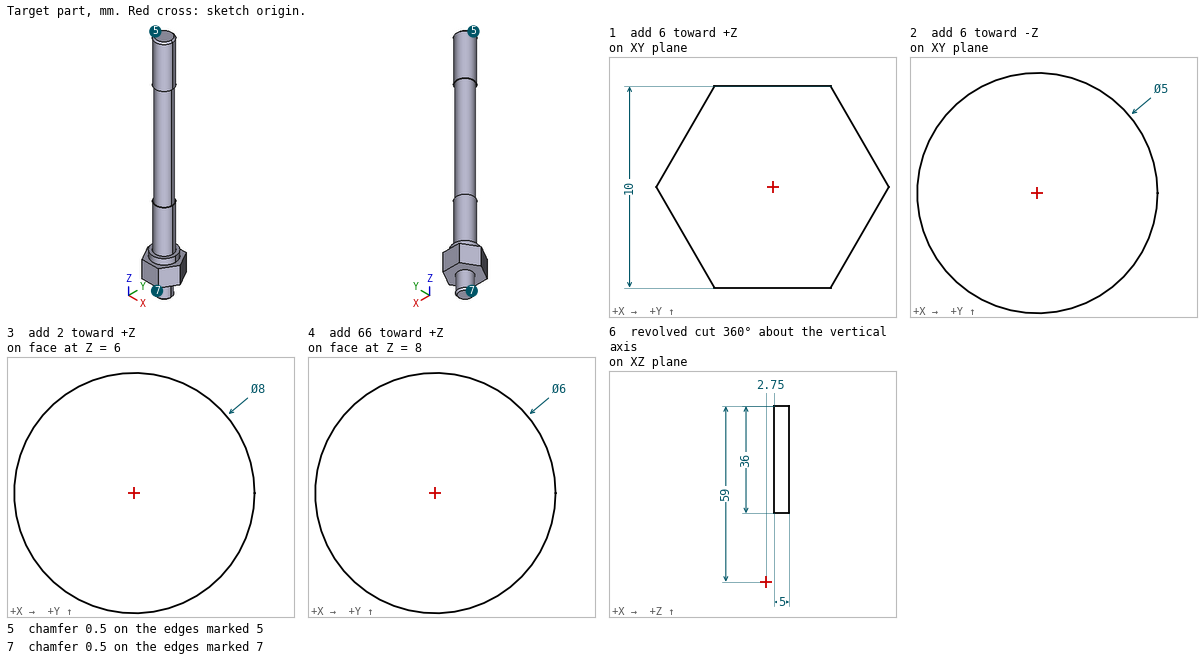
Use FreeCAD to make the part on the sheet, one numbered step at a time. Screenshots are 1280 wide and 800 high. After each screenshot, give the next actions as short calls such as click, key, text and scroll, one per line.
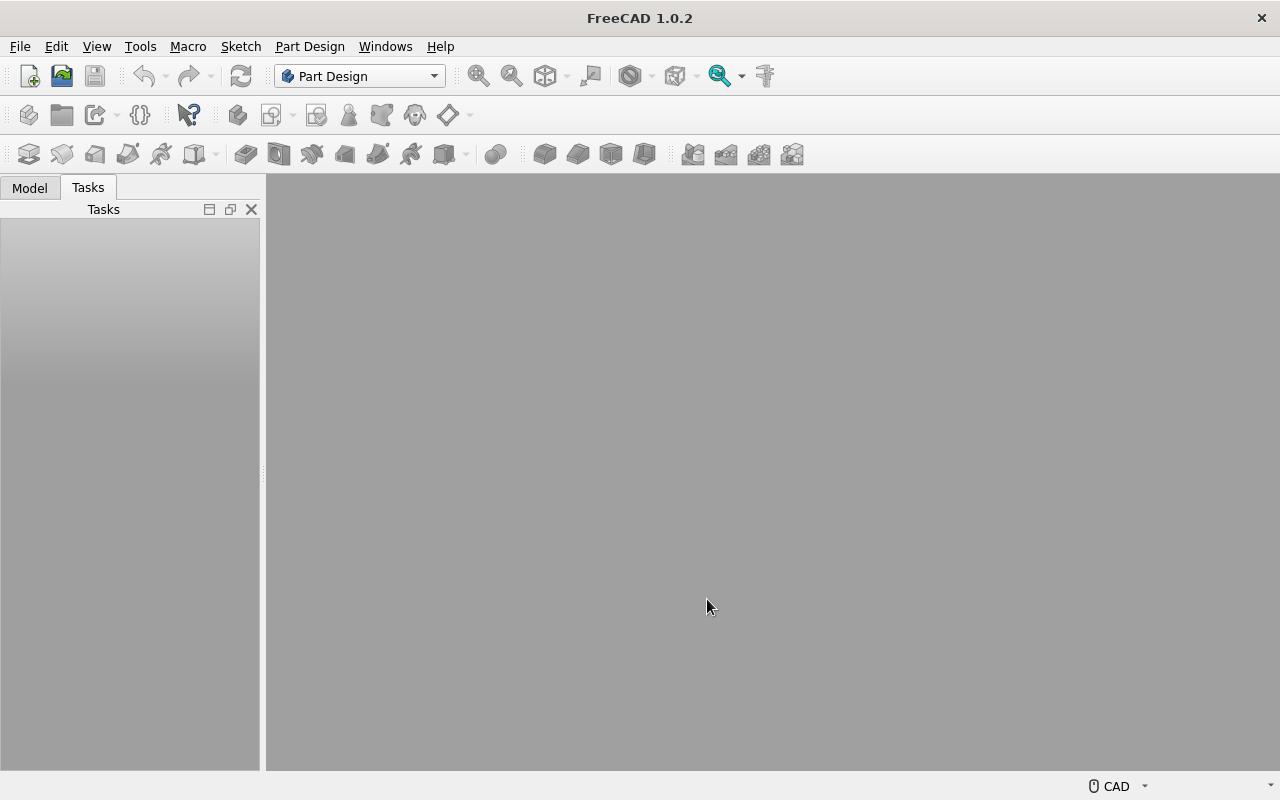
click(29, 76)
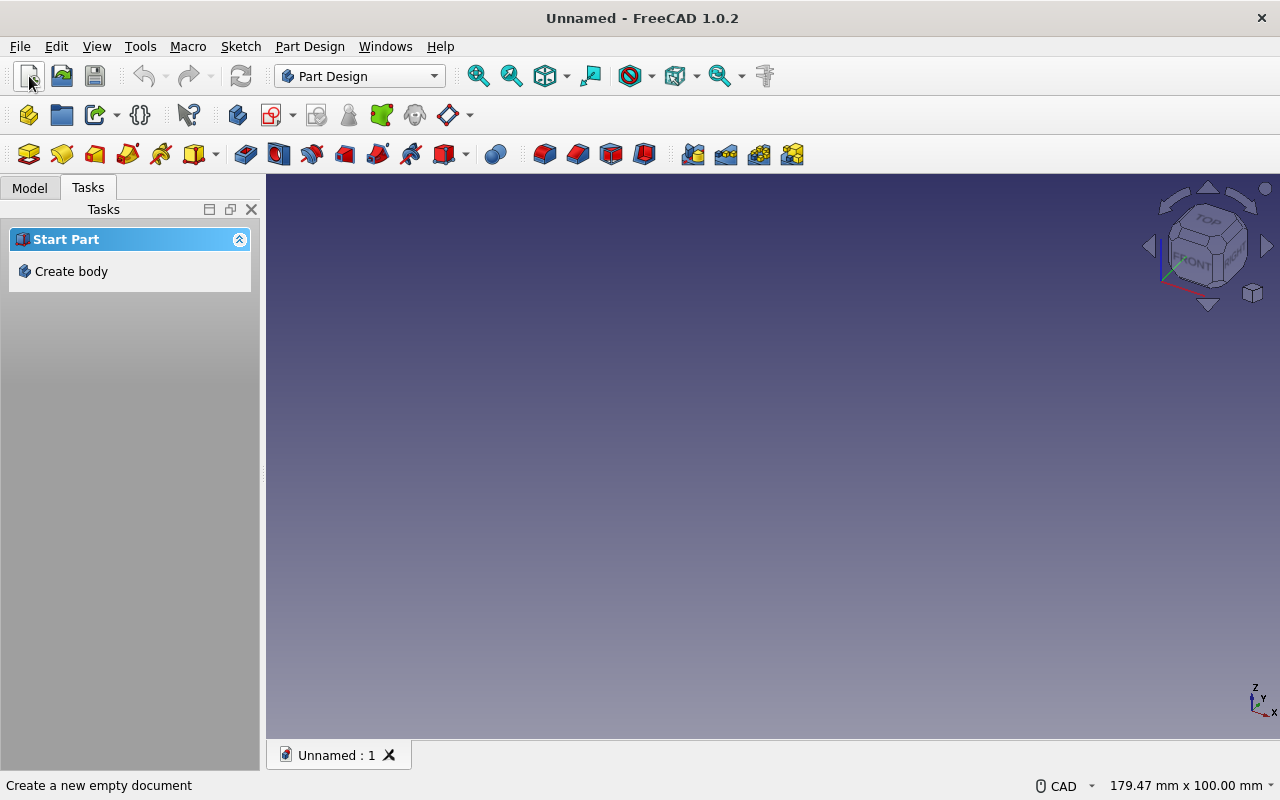
click(270, 116)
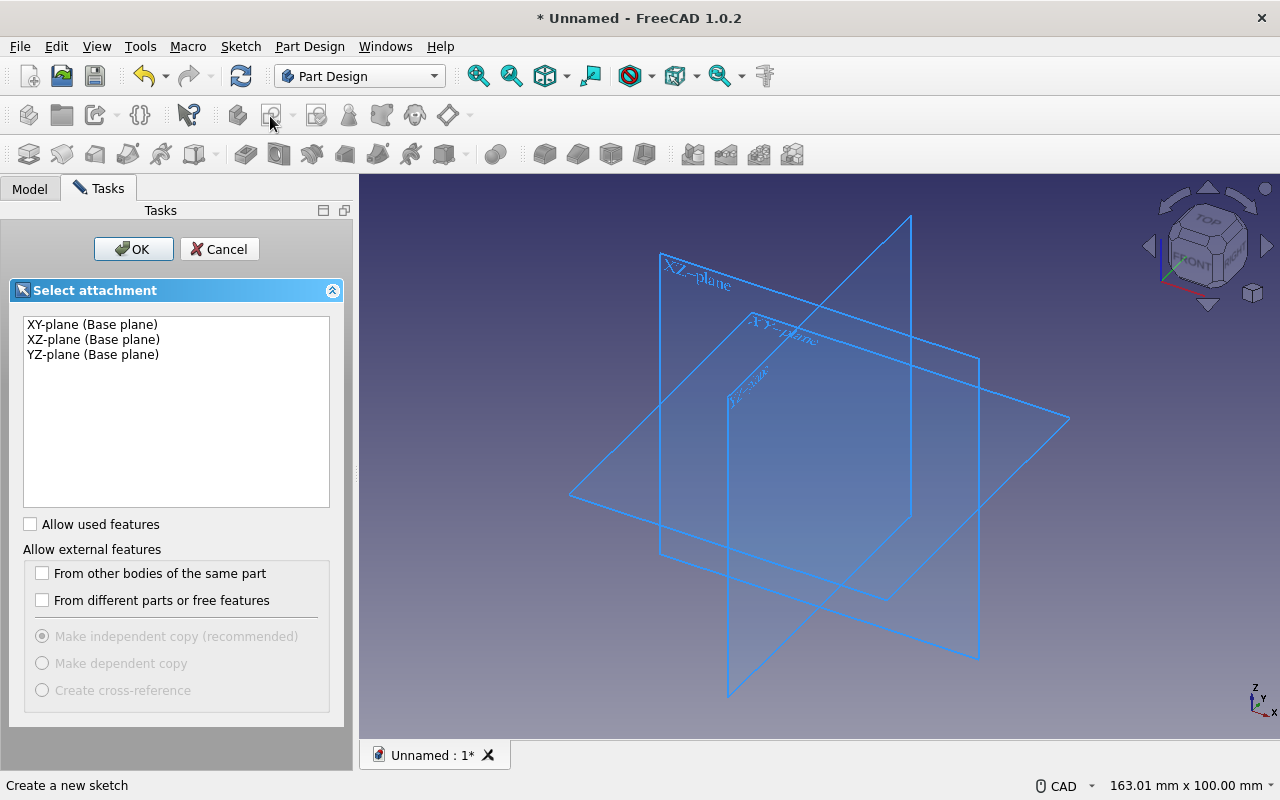
click(84, 324)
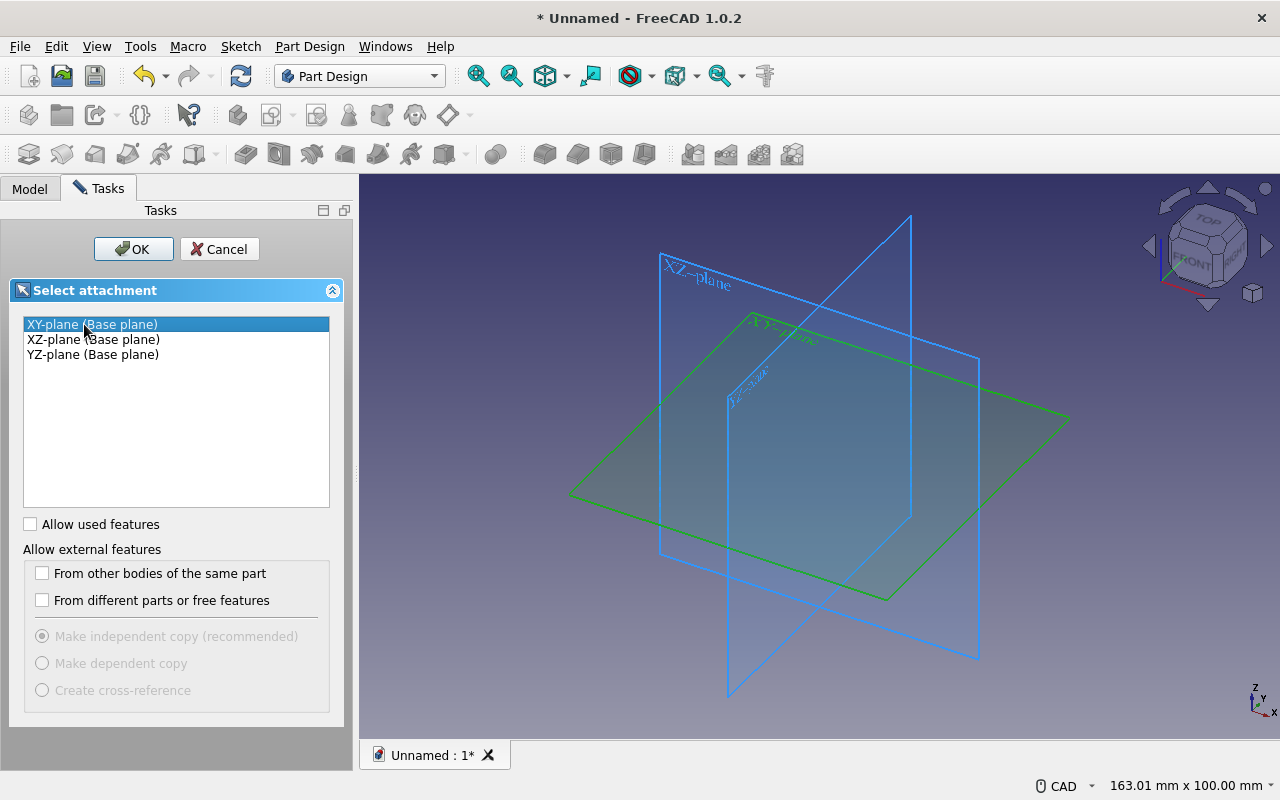
click(134, 249)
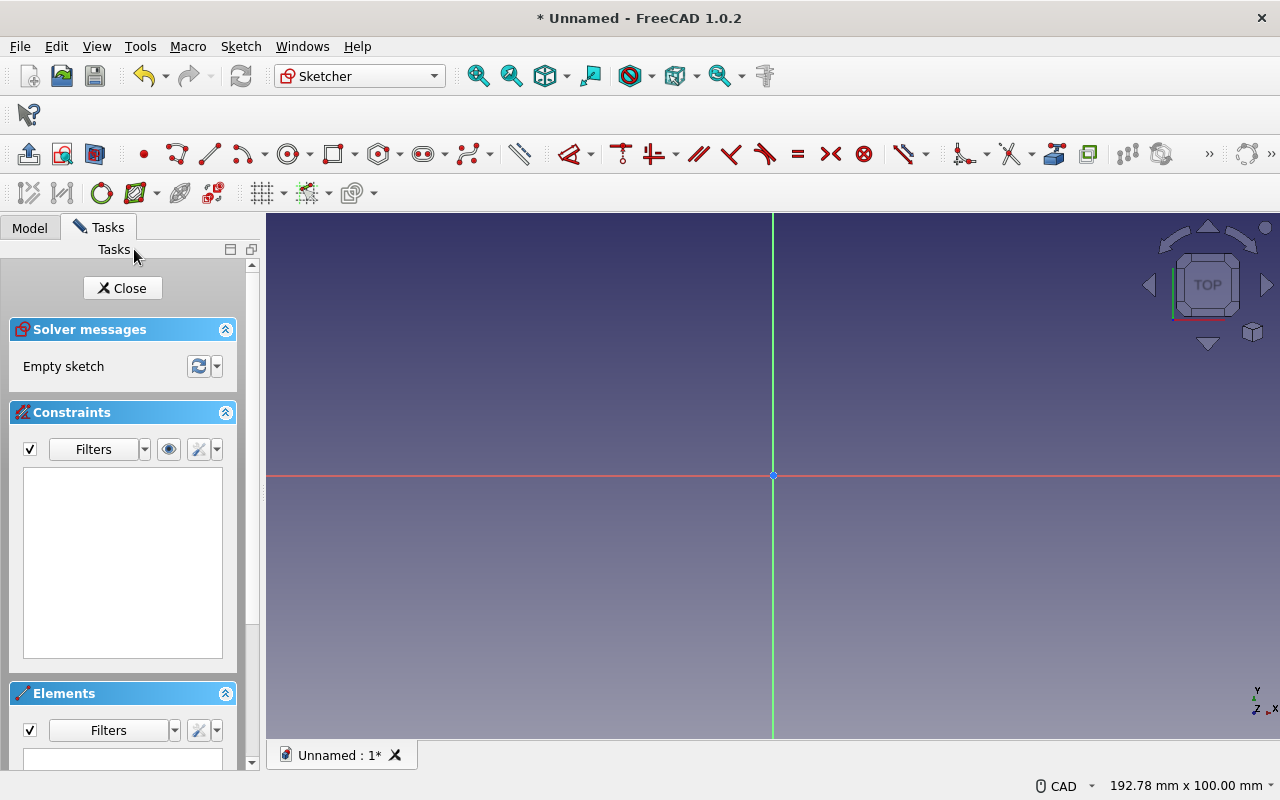
scroll(787, 476, up, 9)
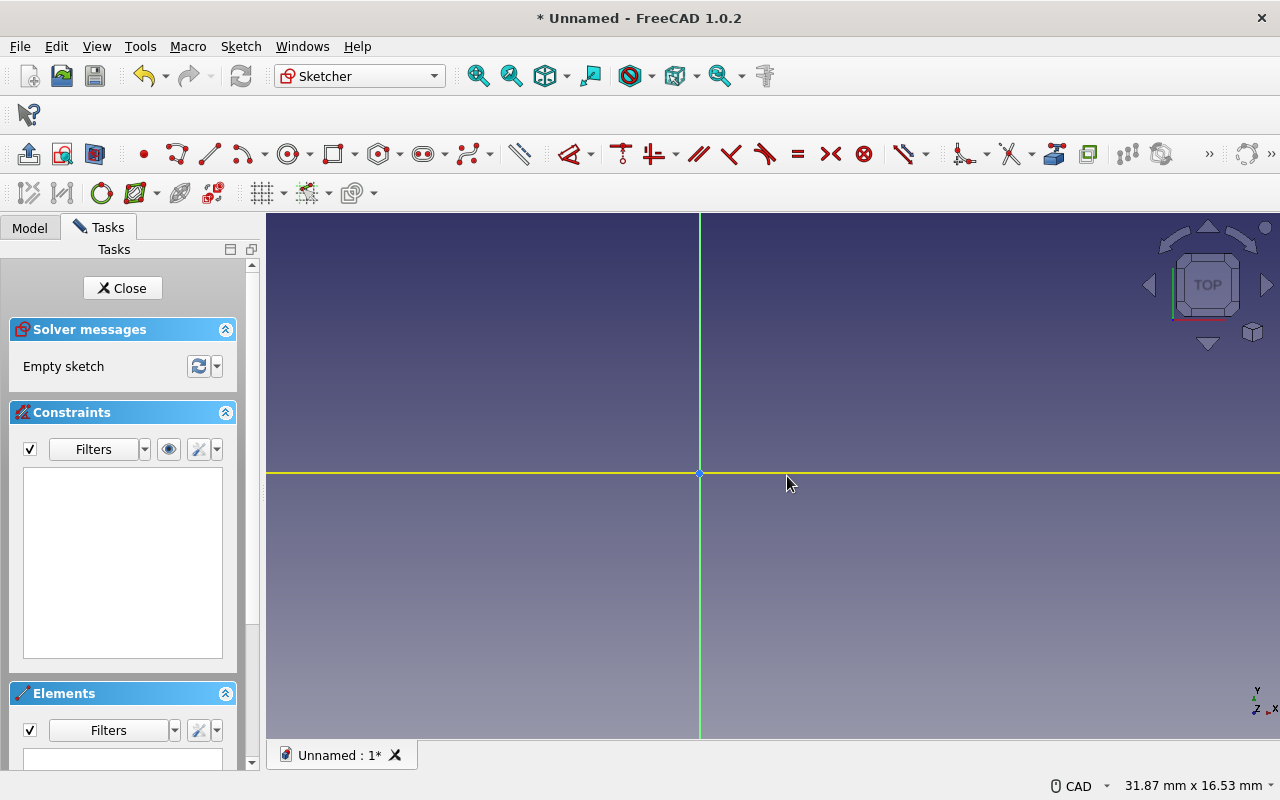
click(378, 154)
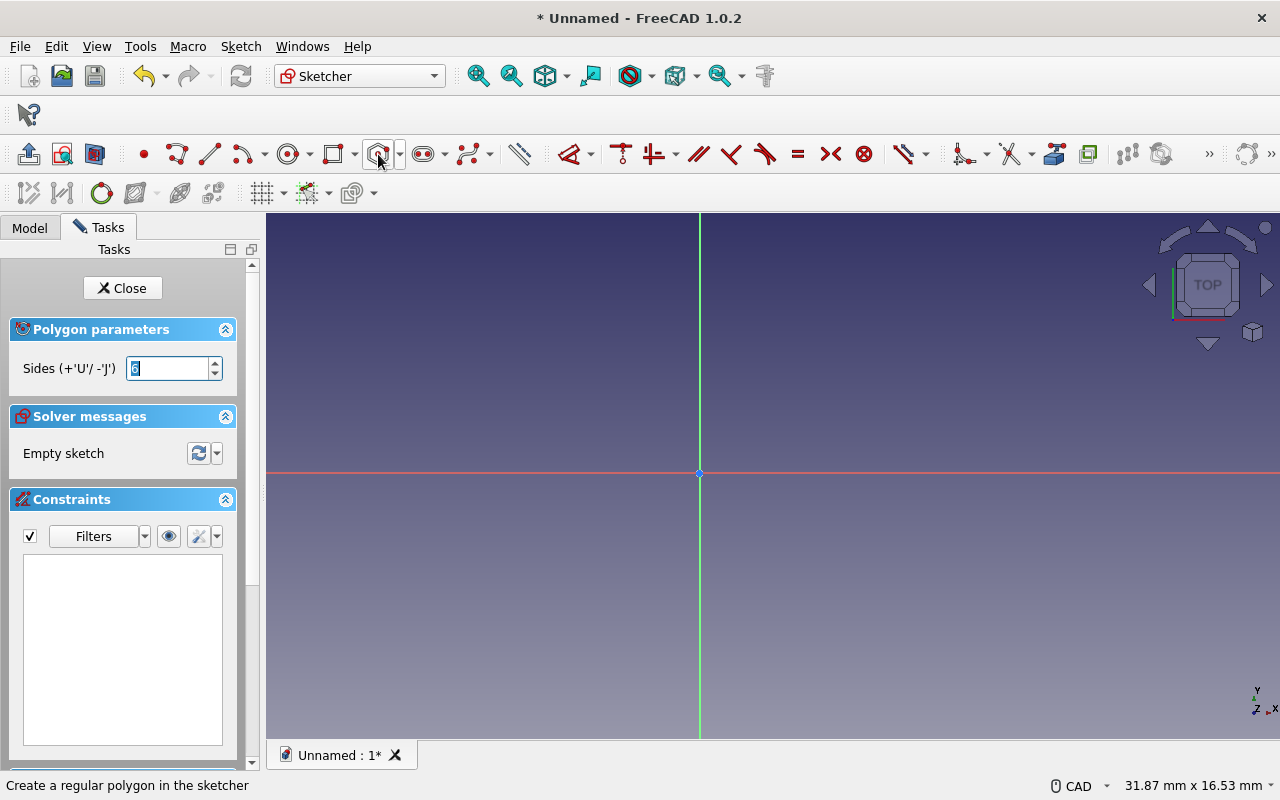
click(700, 473)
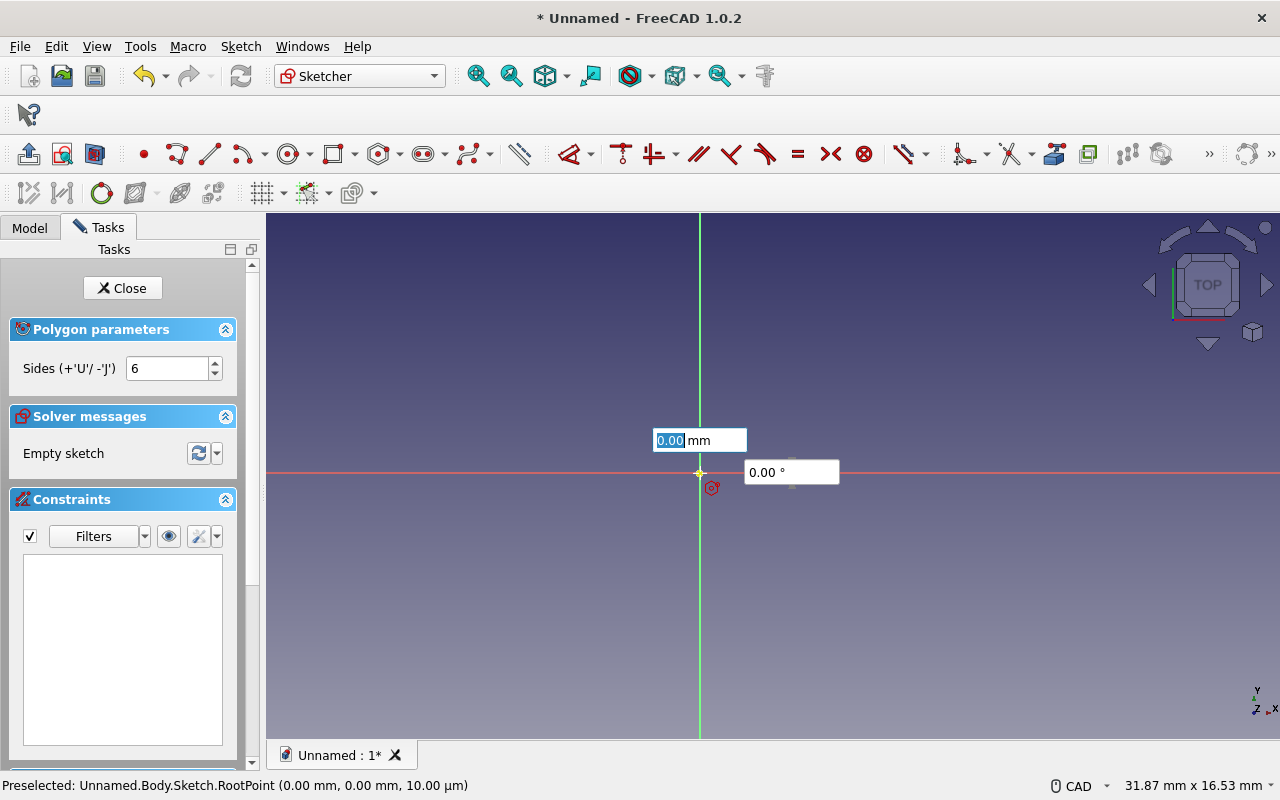
click(883, 473)
key(Escape)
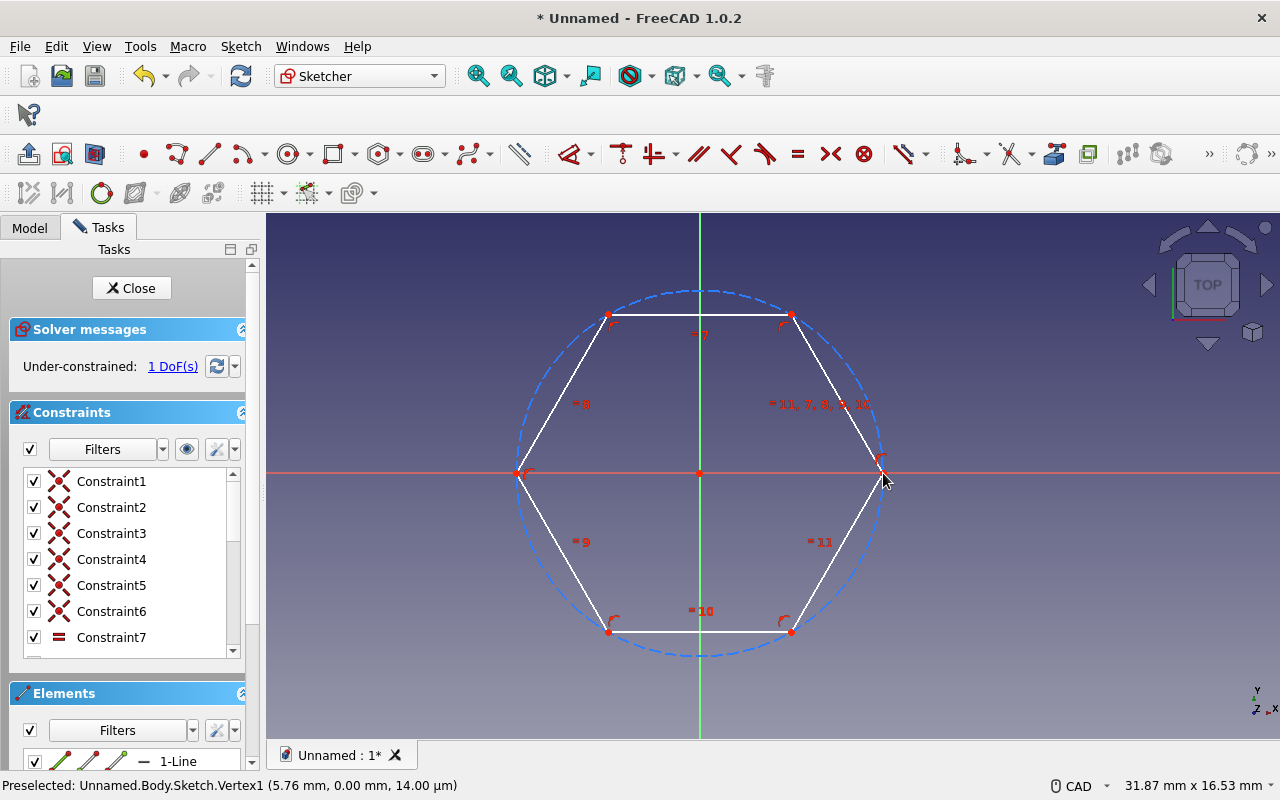
click(608, 632)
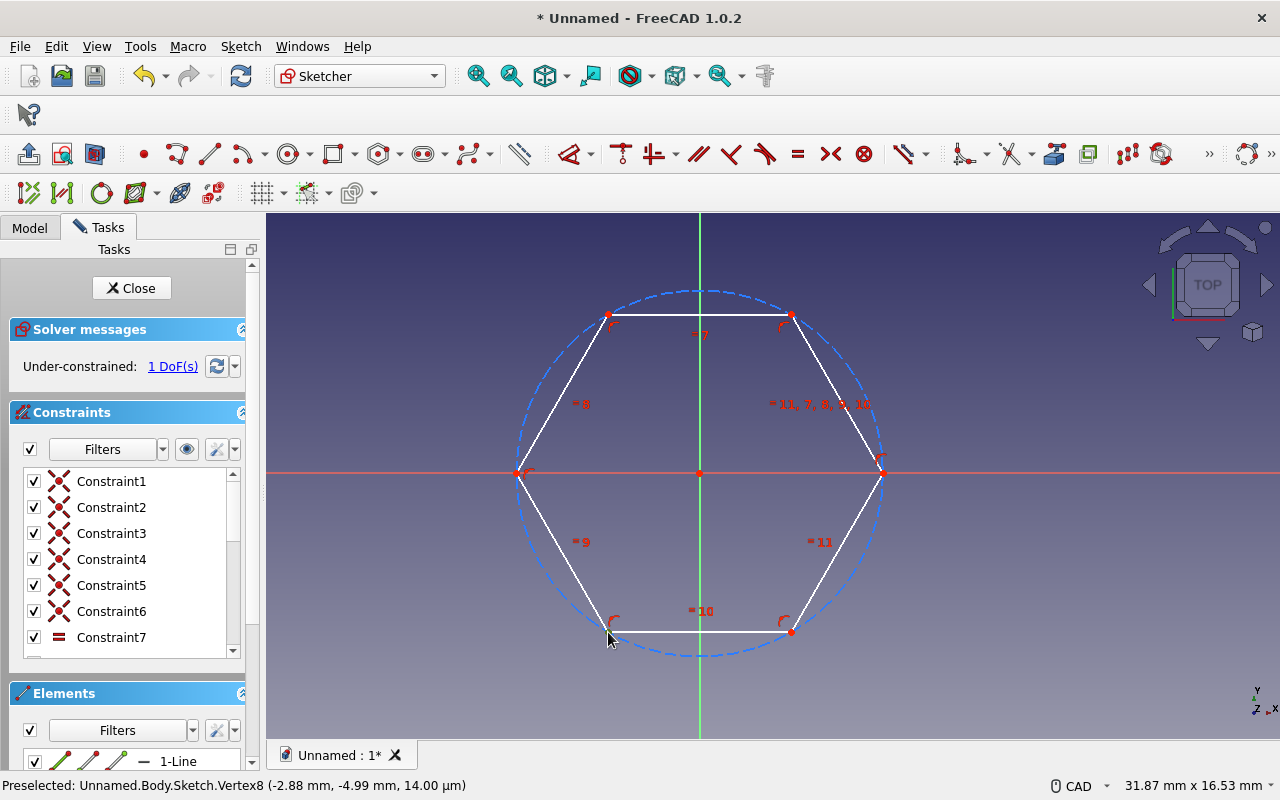
click(791, 315)